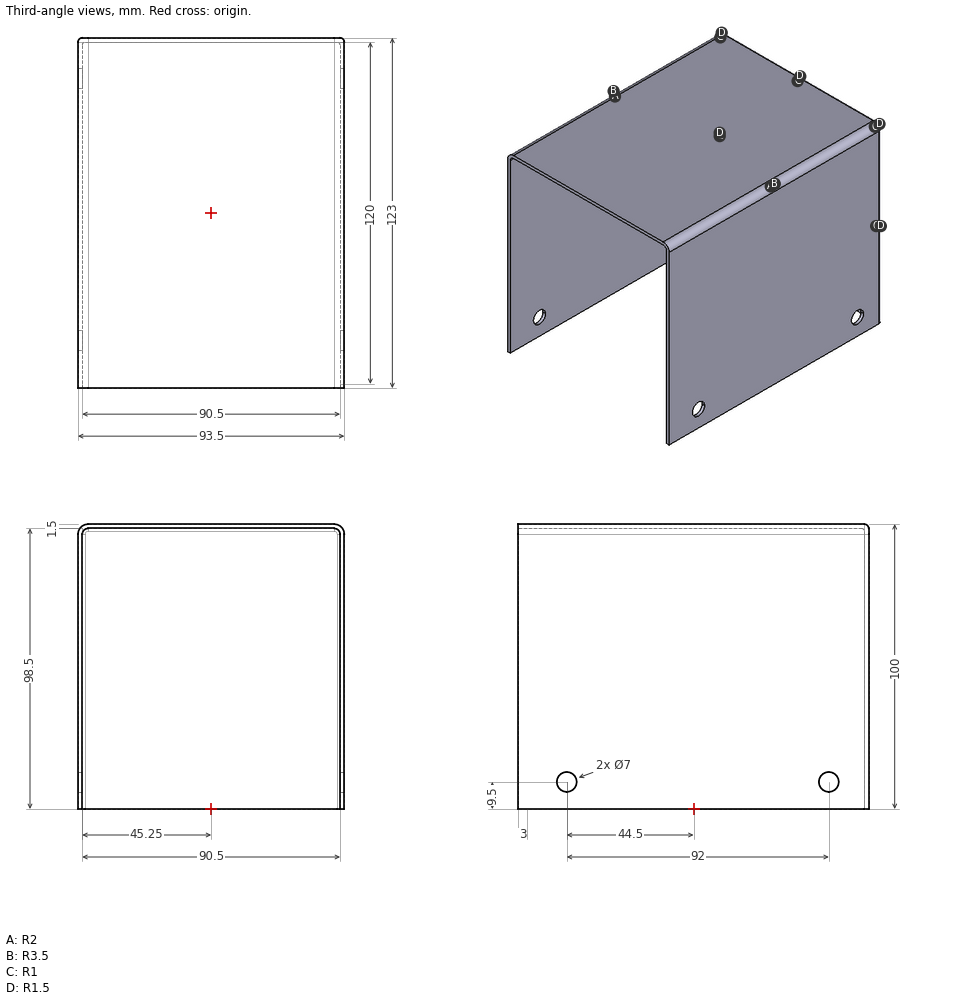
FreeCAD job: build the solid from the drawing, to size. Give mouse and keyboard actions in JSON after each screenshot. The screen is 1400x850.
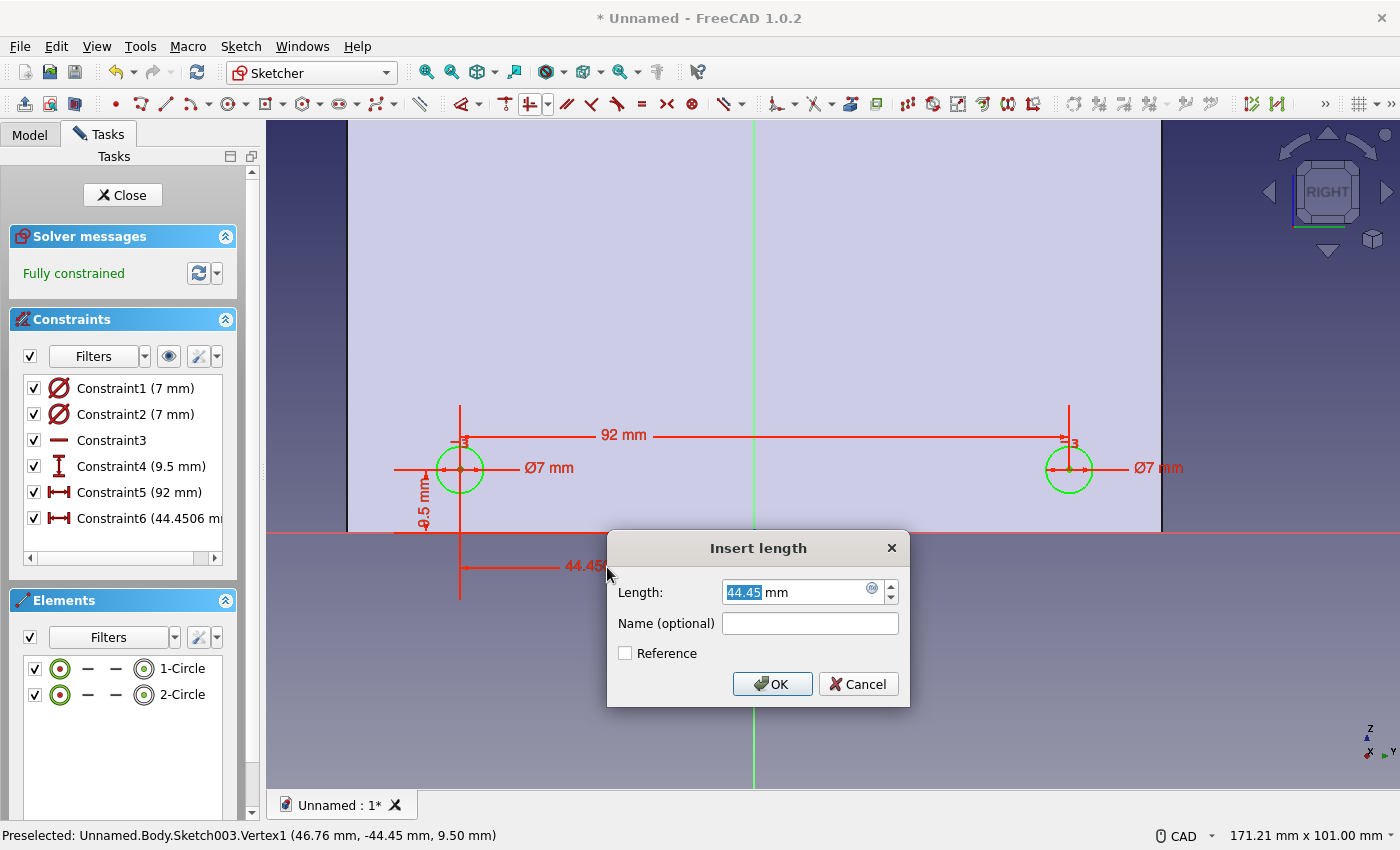
{"action": "type", "text": "44.5"}
{"action": "key", "text": "Return"}
{"action": "key", "text": "Escape"}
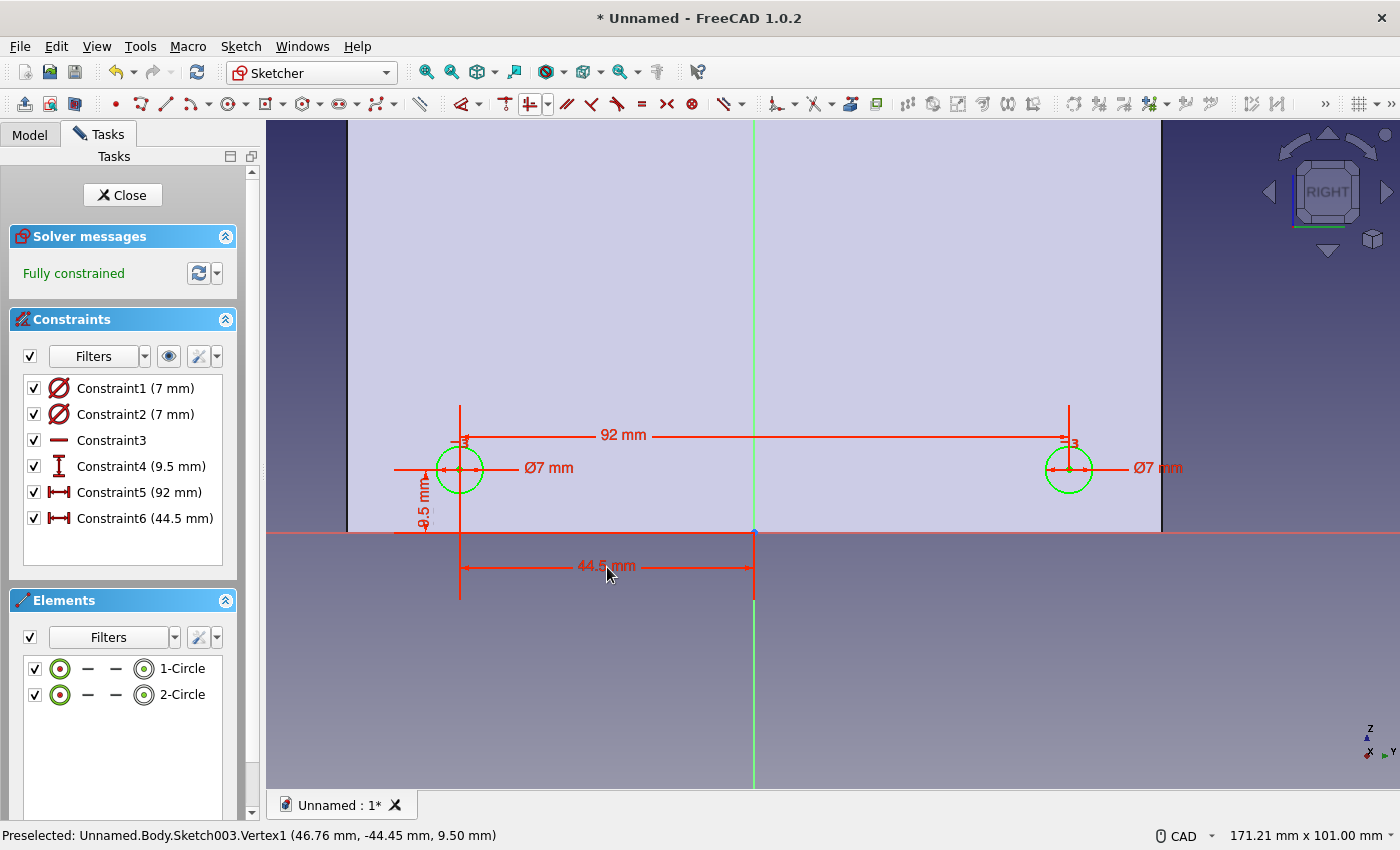
{"action": "left_click", "coordinate": [123, 195]}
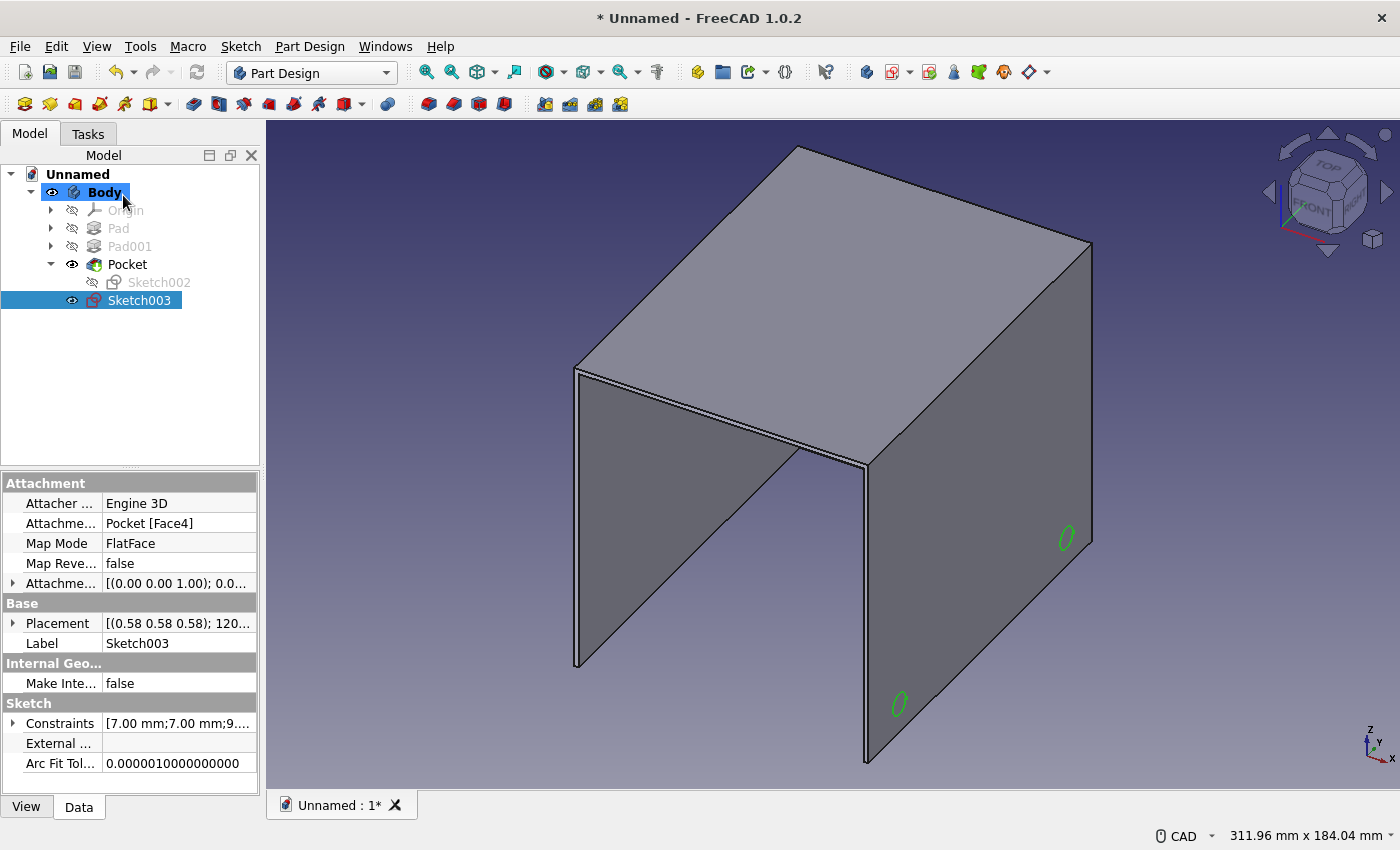
{"action": "left_click", "coordinate": [194, 104]}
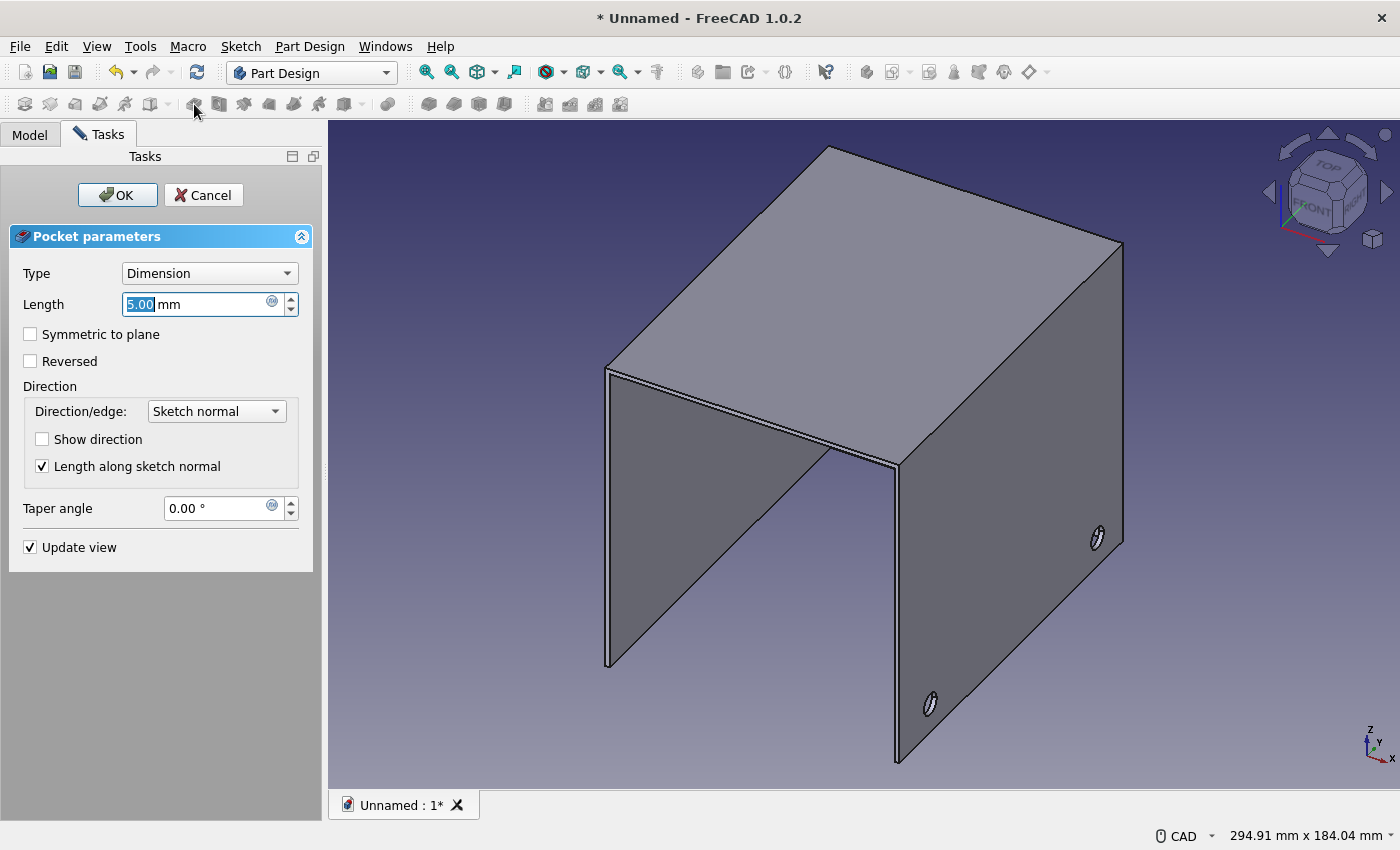
{"action": "left_click", "coordinate": [210, 274]}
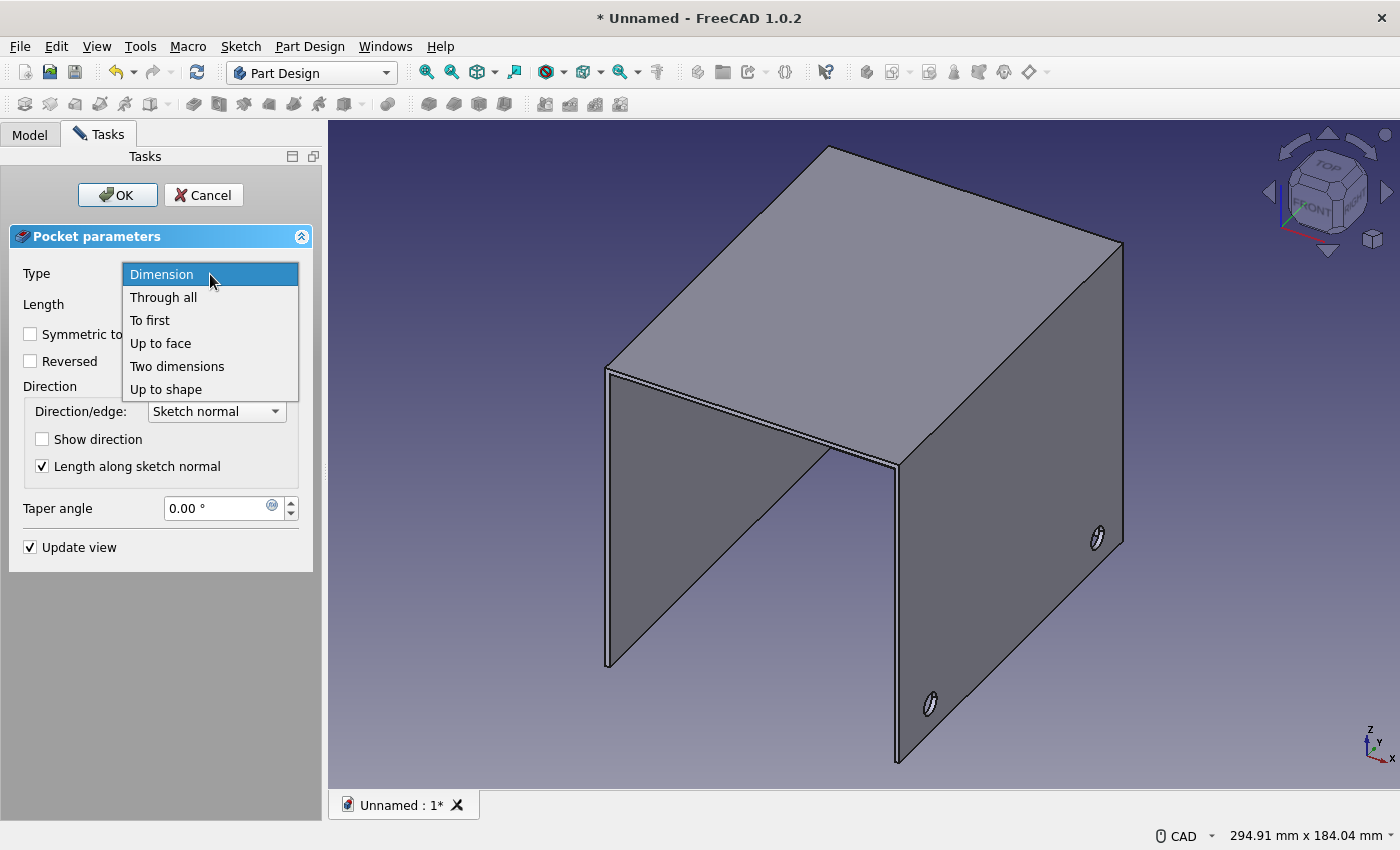
{"action": "left_click", "coordinate": [208, 298]}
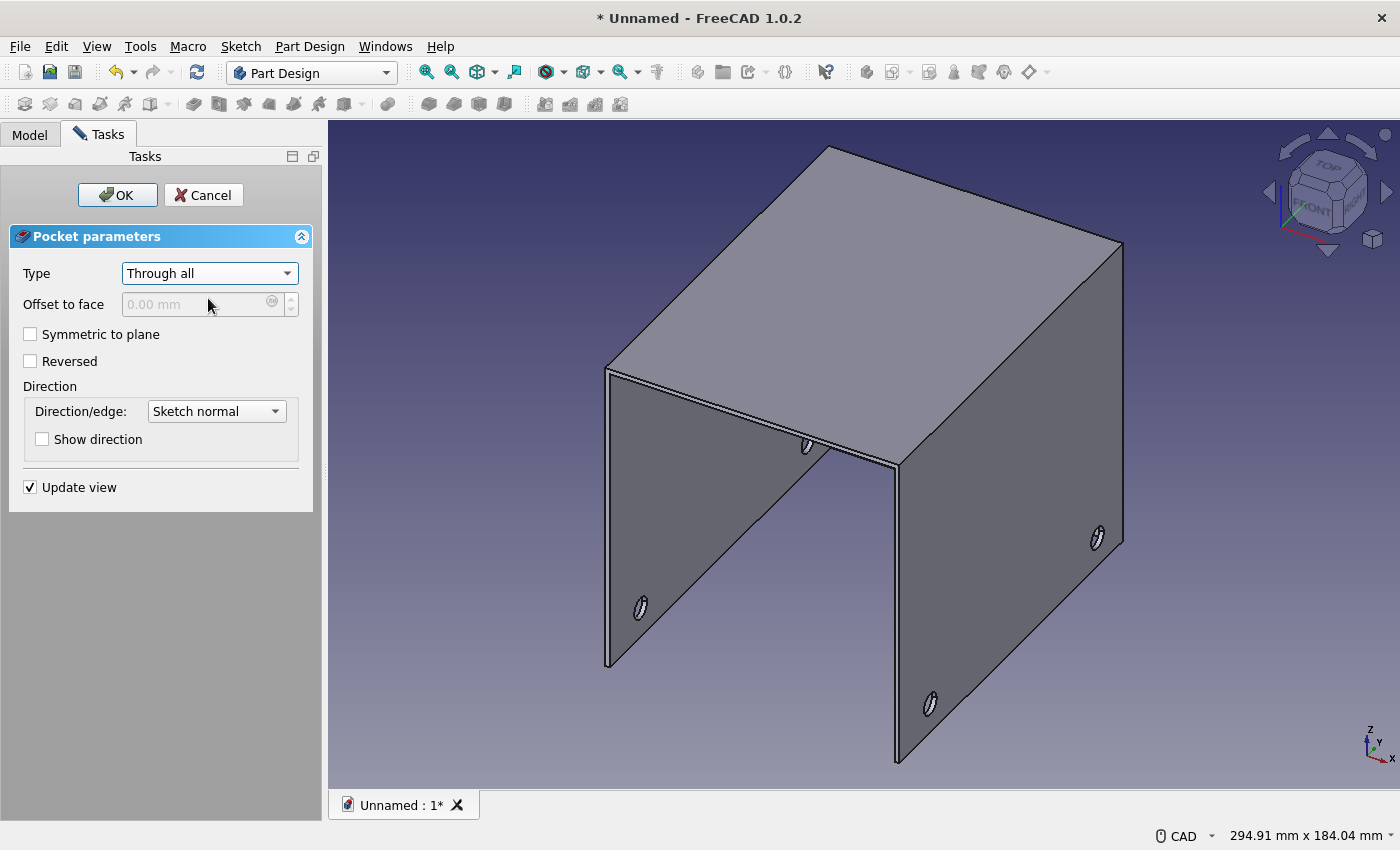
{"action": "left_click", "coordinate": [118, 195]}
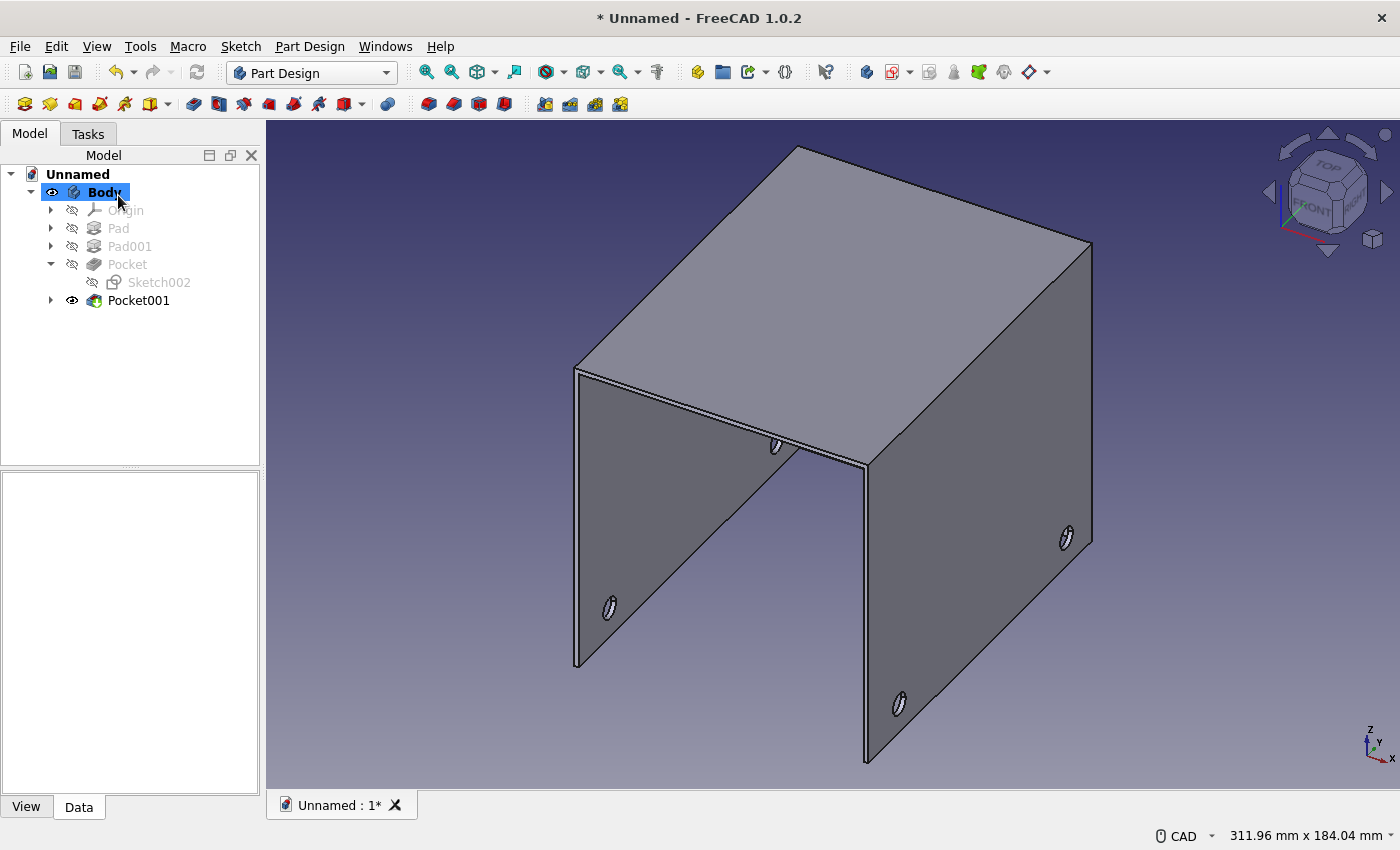
{"action": "key", "text": "0"}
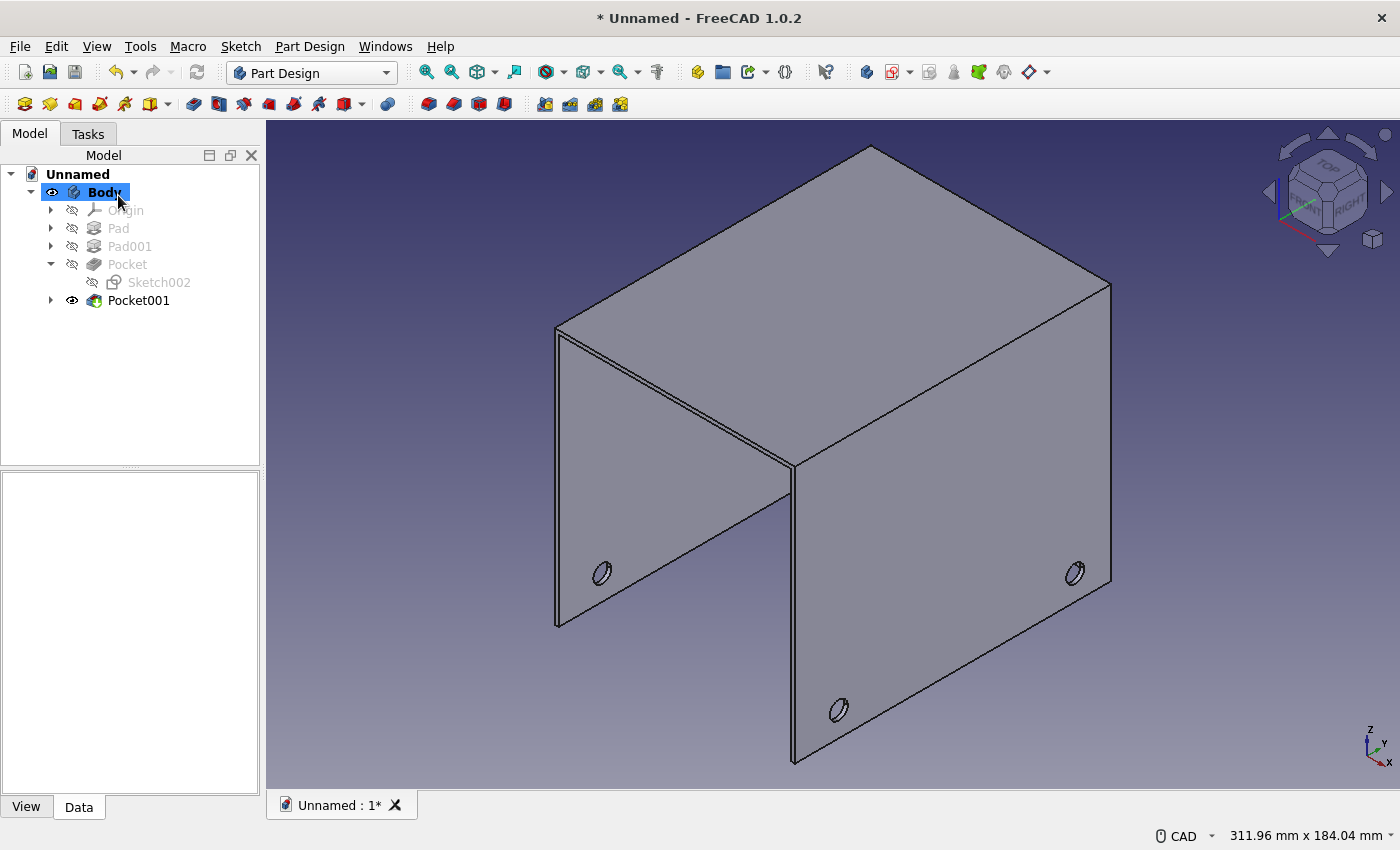
{"action": "key", "text": "2"}